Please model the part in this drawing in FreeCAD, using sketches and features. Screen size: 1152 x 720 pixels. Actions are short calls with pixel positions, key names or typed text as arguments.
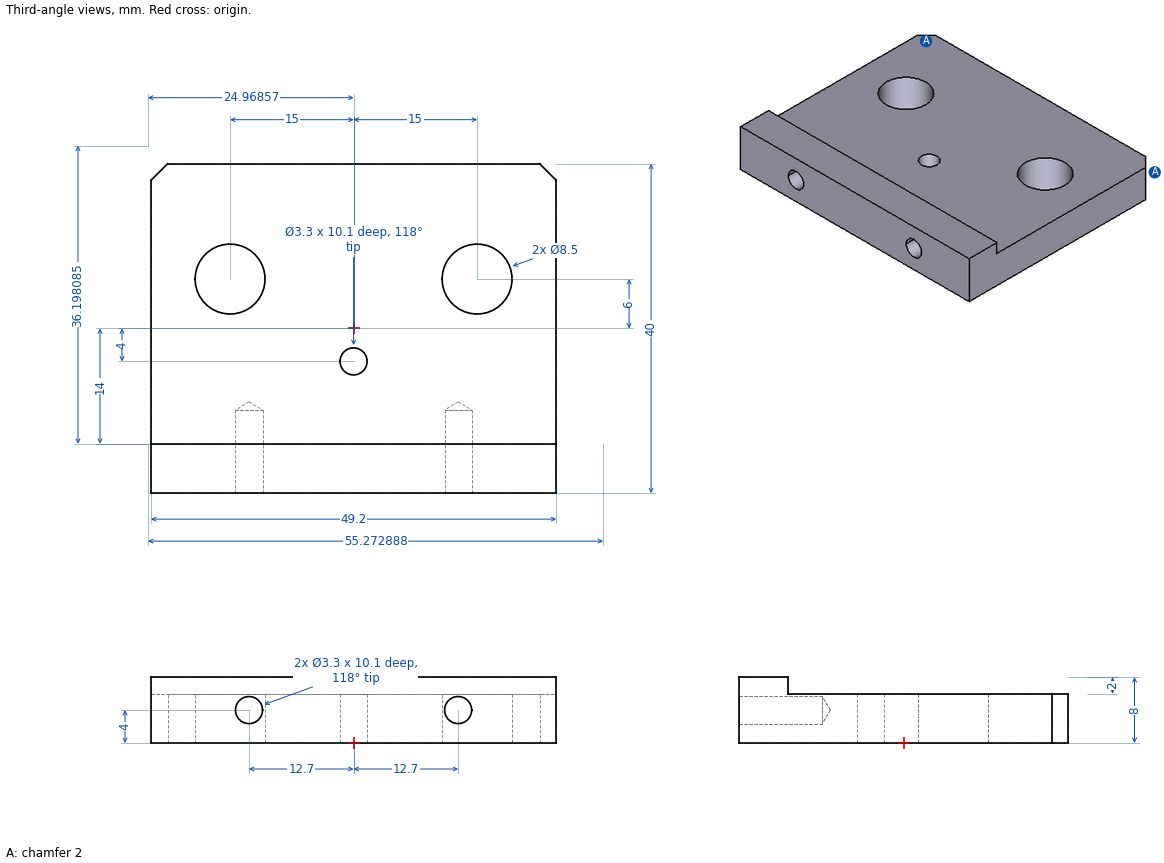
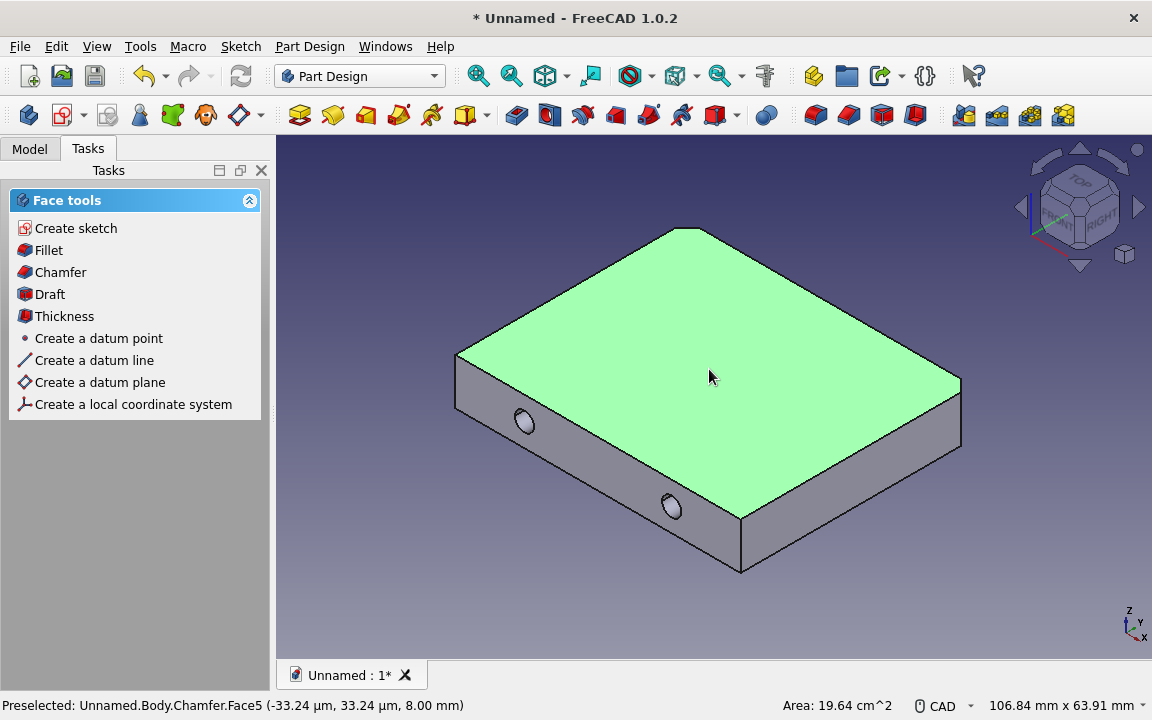
click(62, 116)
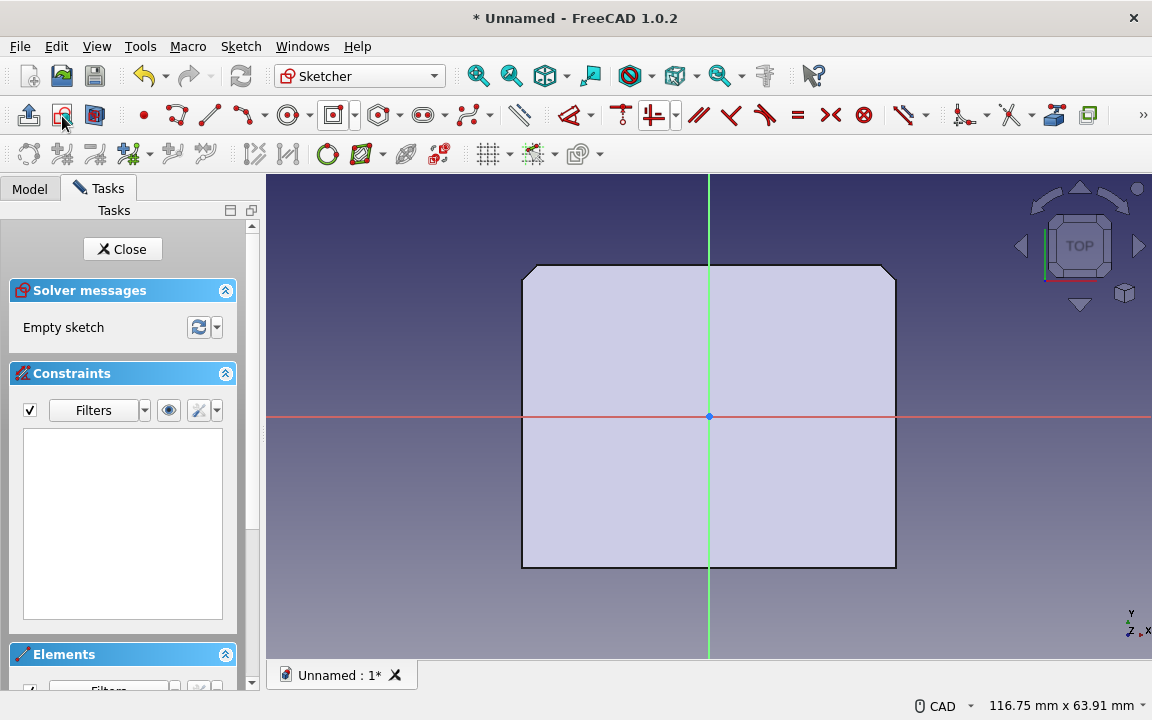
click(354, 116)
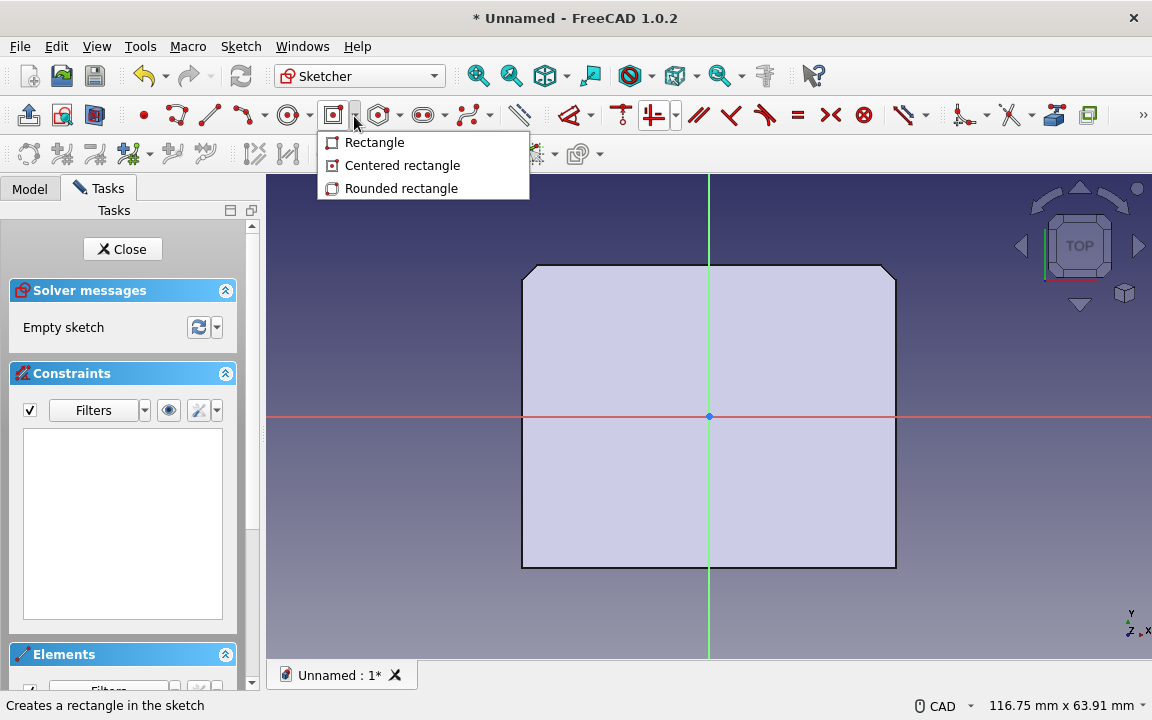
click(424, 142)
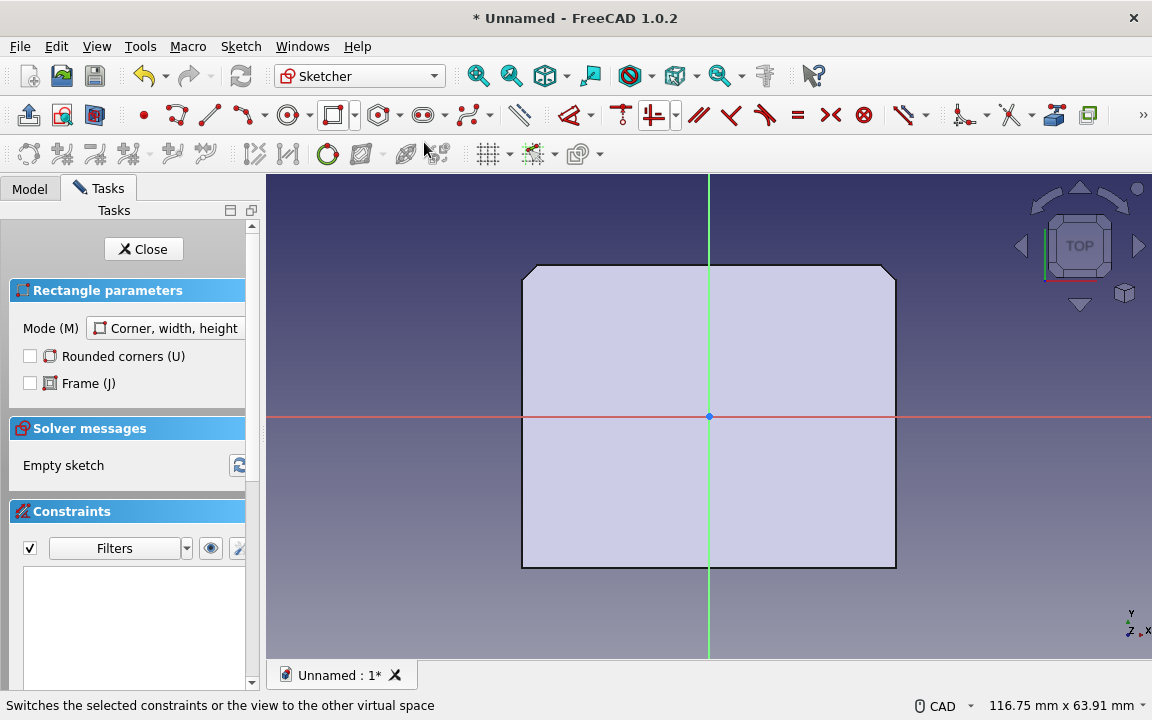
click(520, 248)
click(939, 523)
key(Escape)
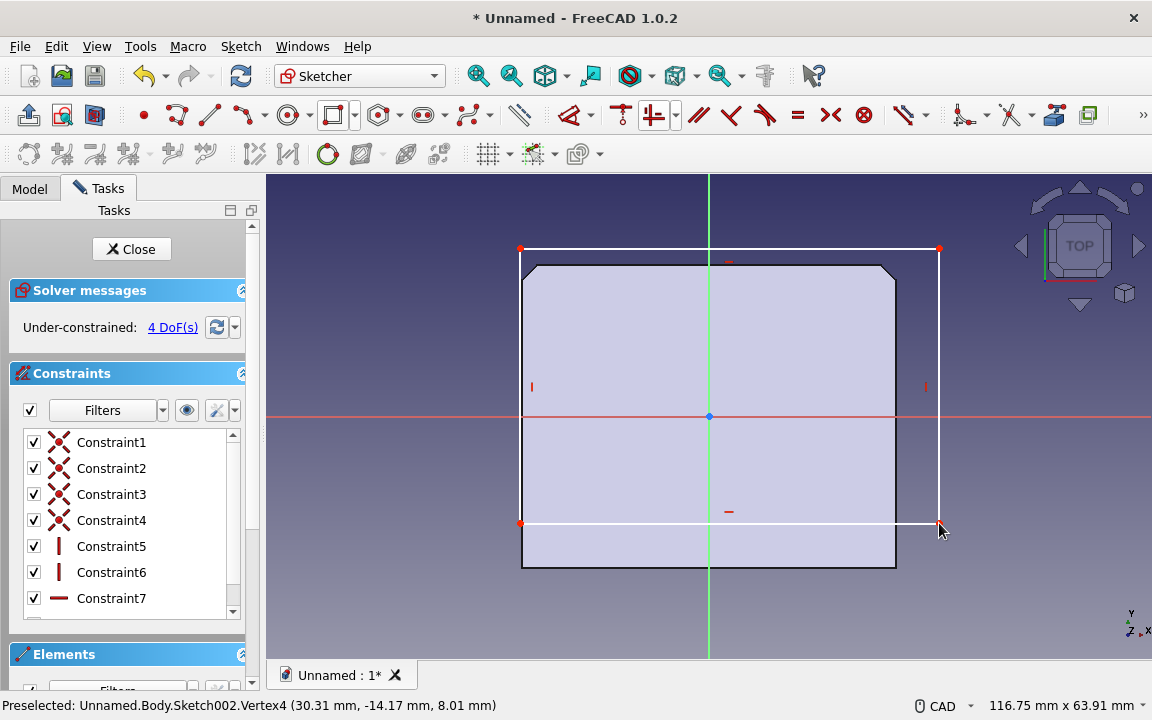
key(d)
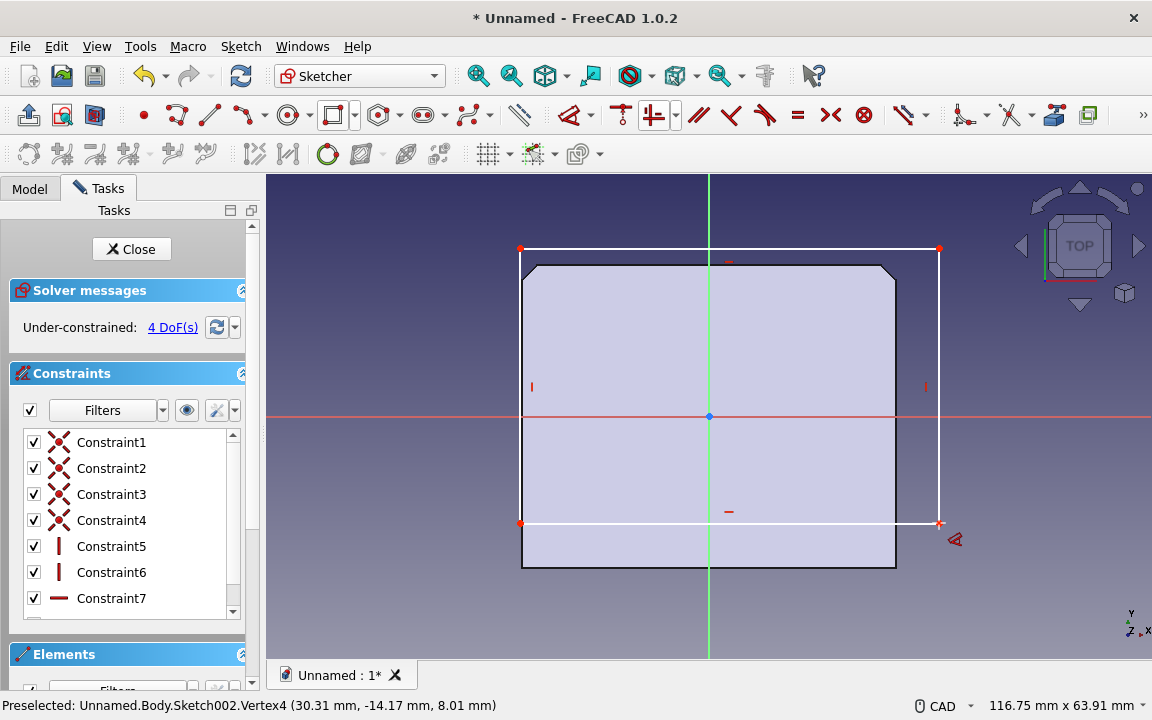
click(520, 524)
click(486, 470)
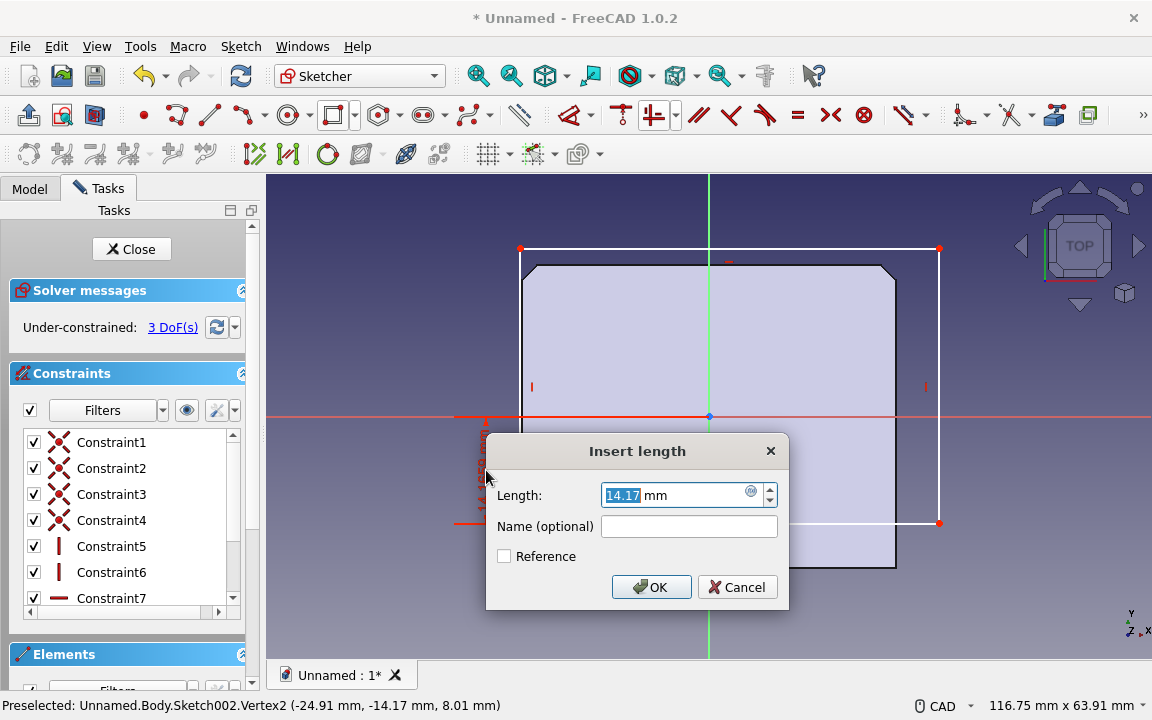
text(14)
key(Return)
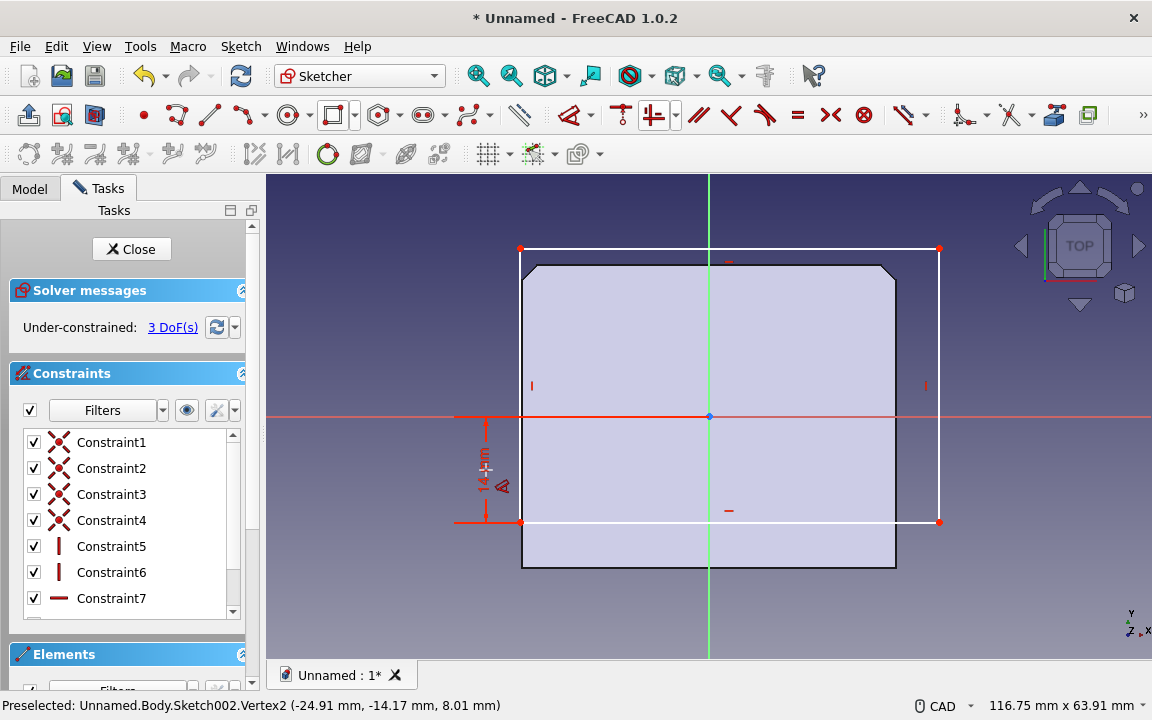
click(520, 331)
click(486, 386)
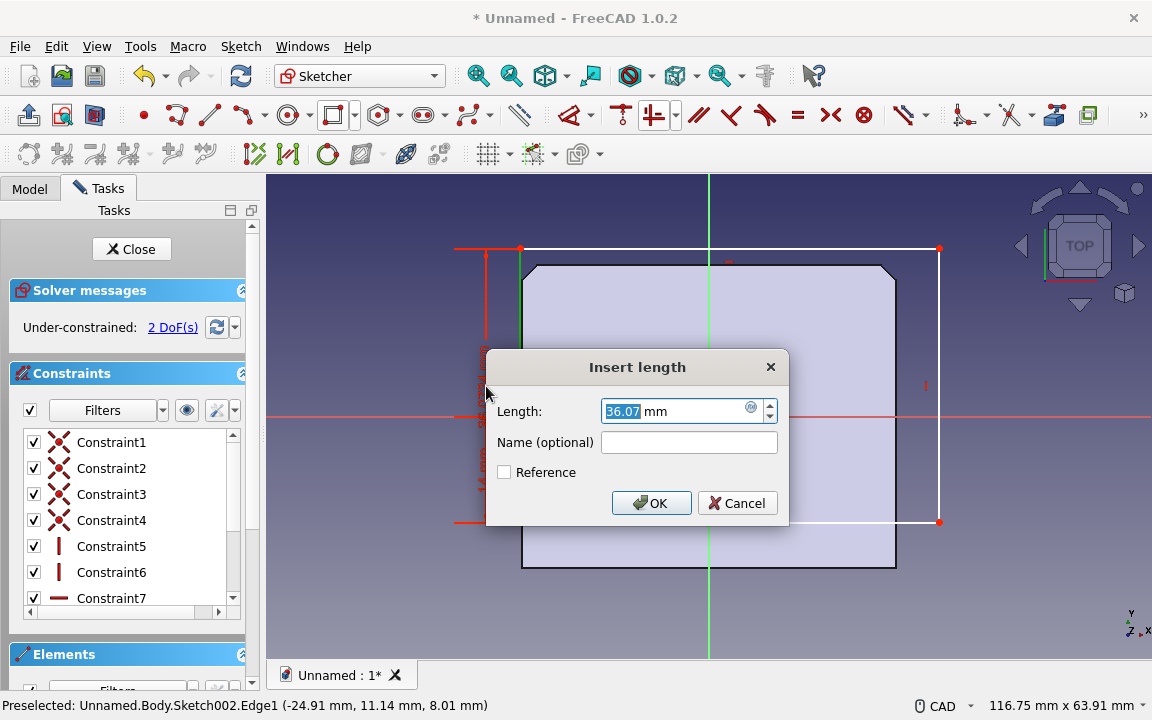
text(36.198085)
key(Return)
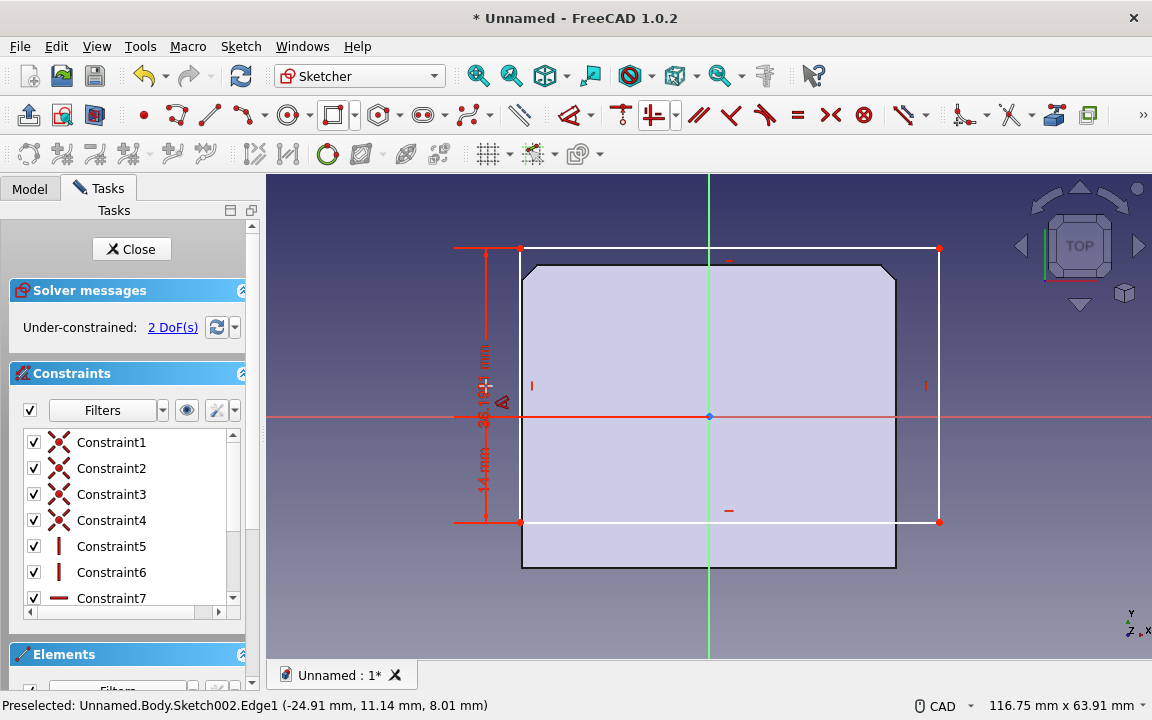
click(646, 523)
click(730, 557)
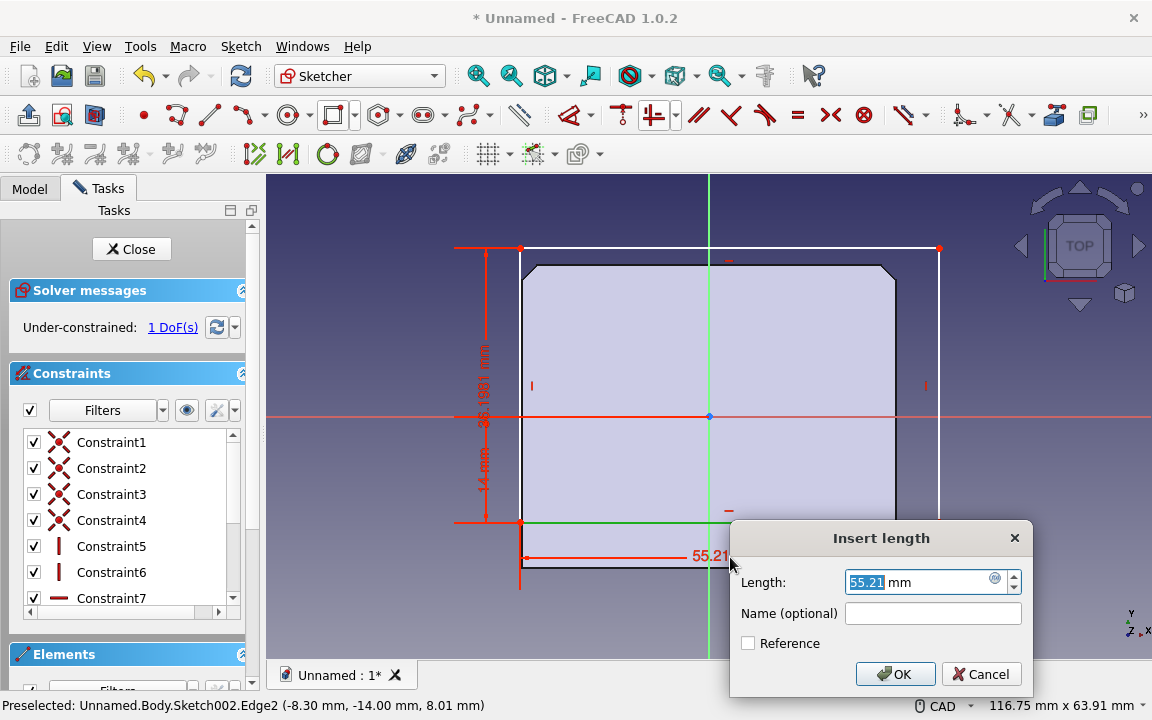
text(55.272888)
key(Return)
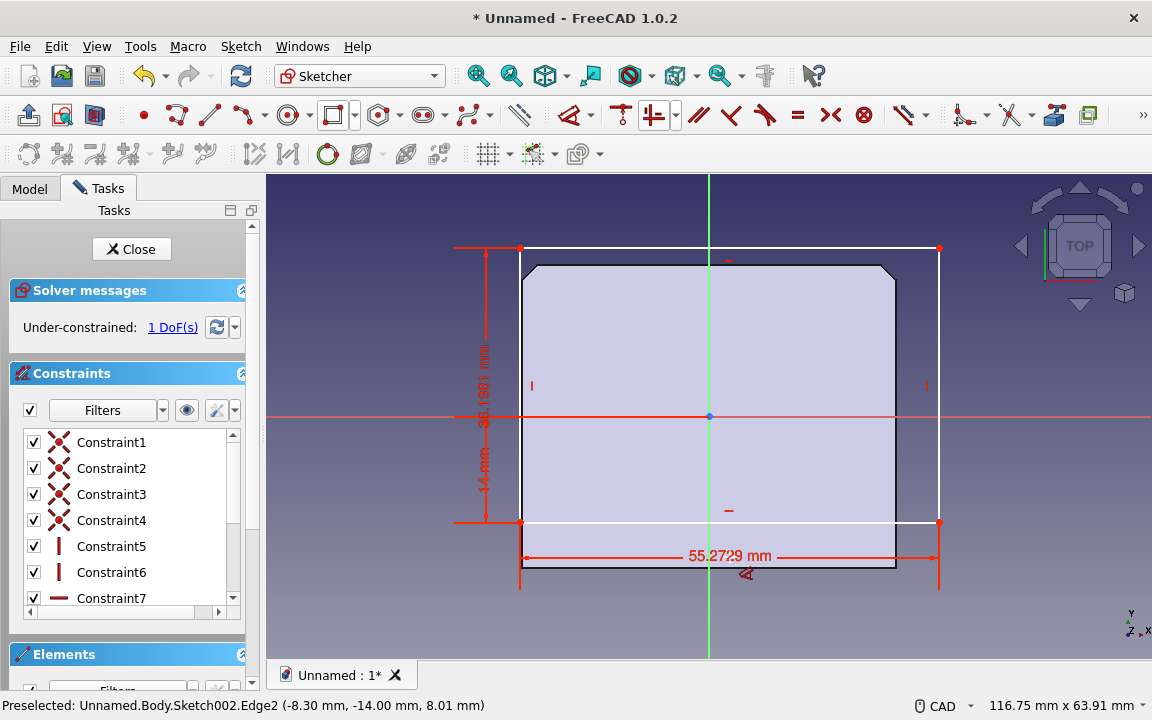
click(520, 248)
click(614, 214)